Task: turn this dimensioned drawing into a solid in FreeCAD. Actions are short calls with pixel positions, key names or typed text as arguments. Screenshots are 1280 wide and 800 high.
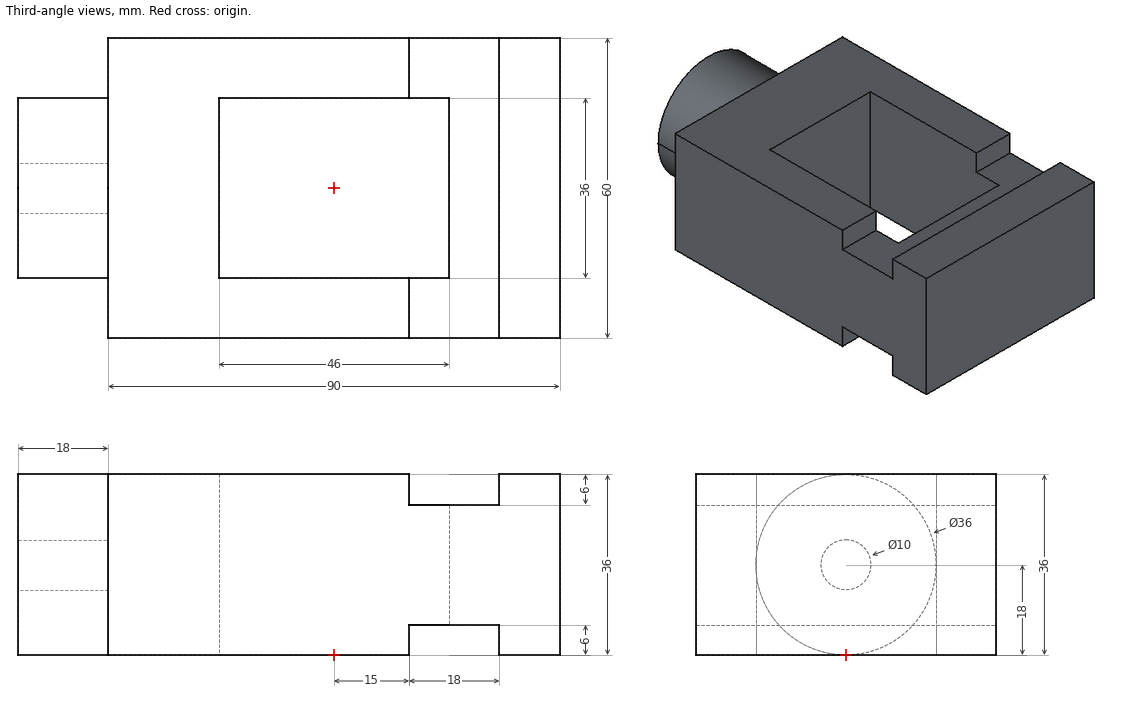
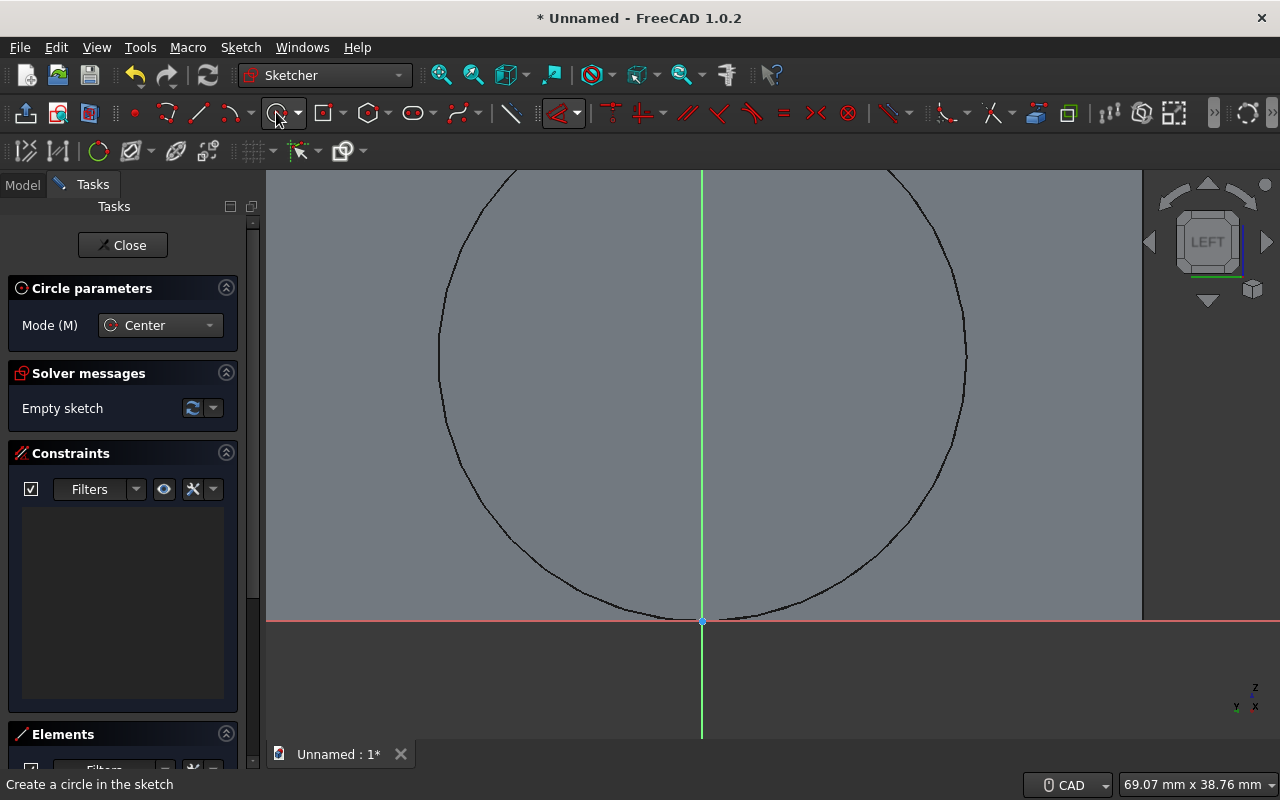
click(702, 357)
click(754, 305)
key(Escape)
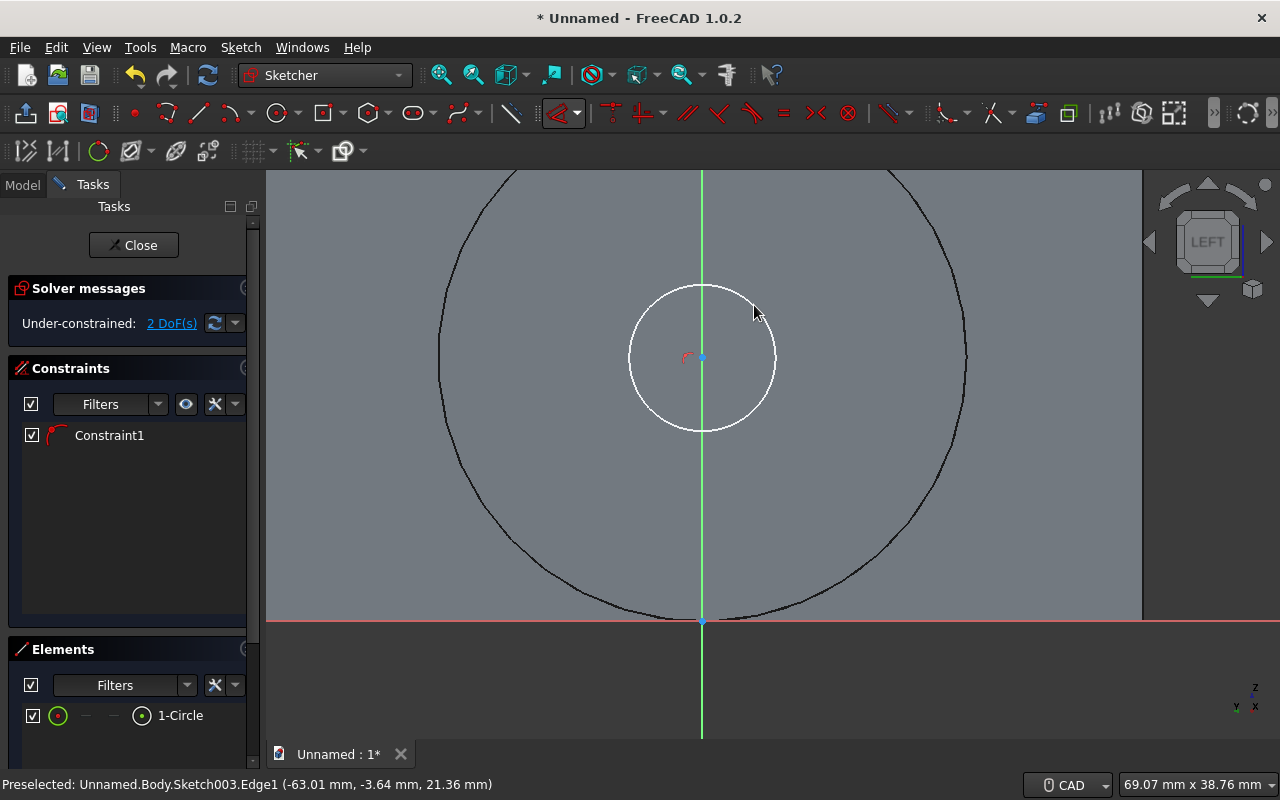
click(754, 306)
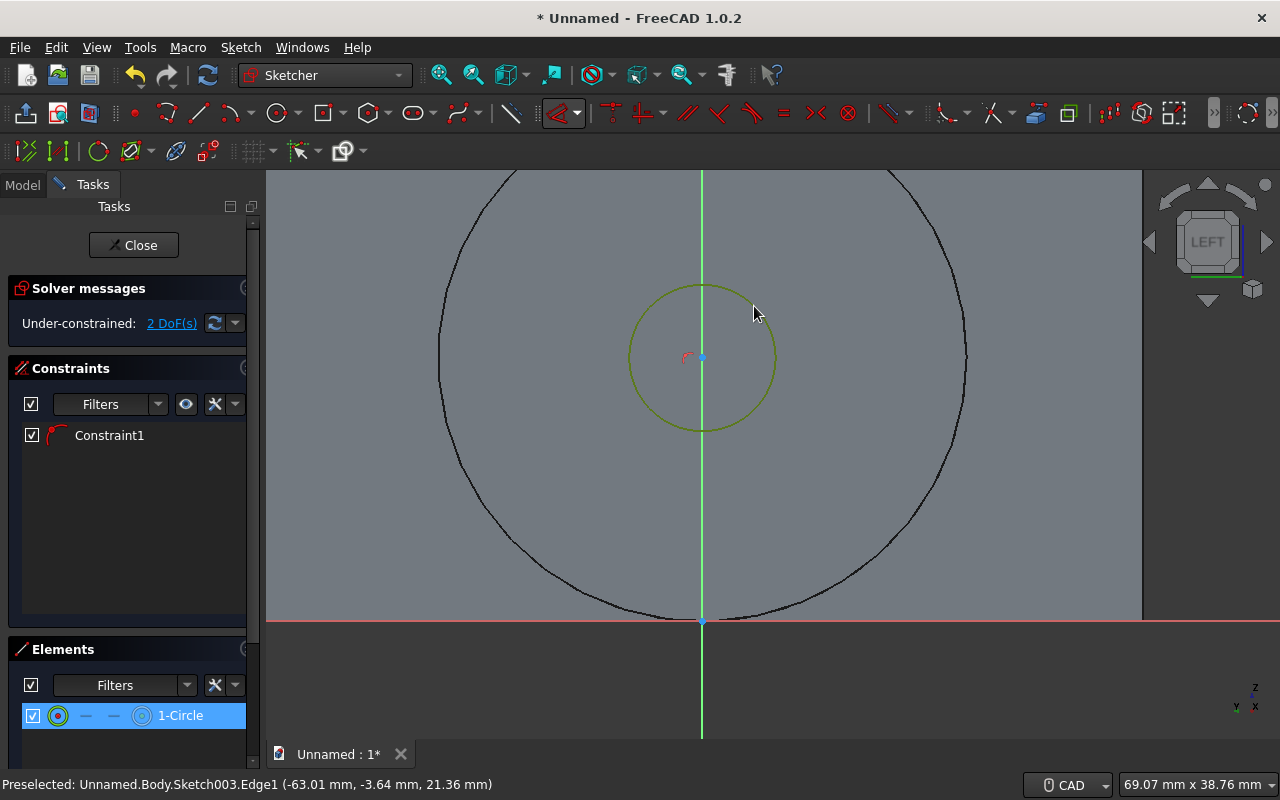
click(580, 114)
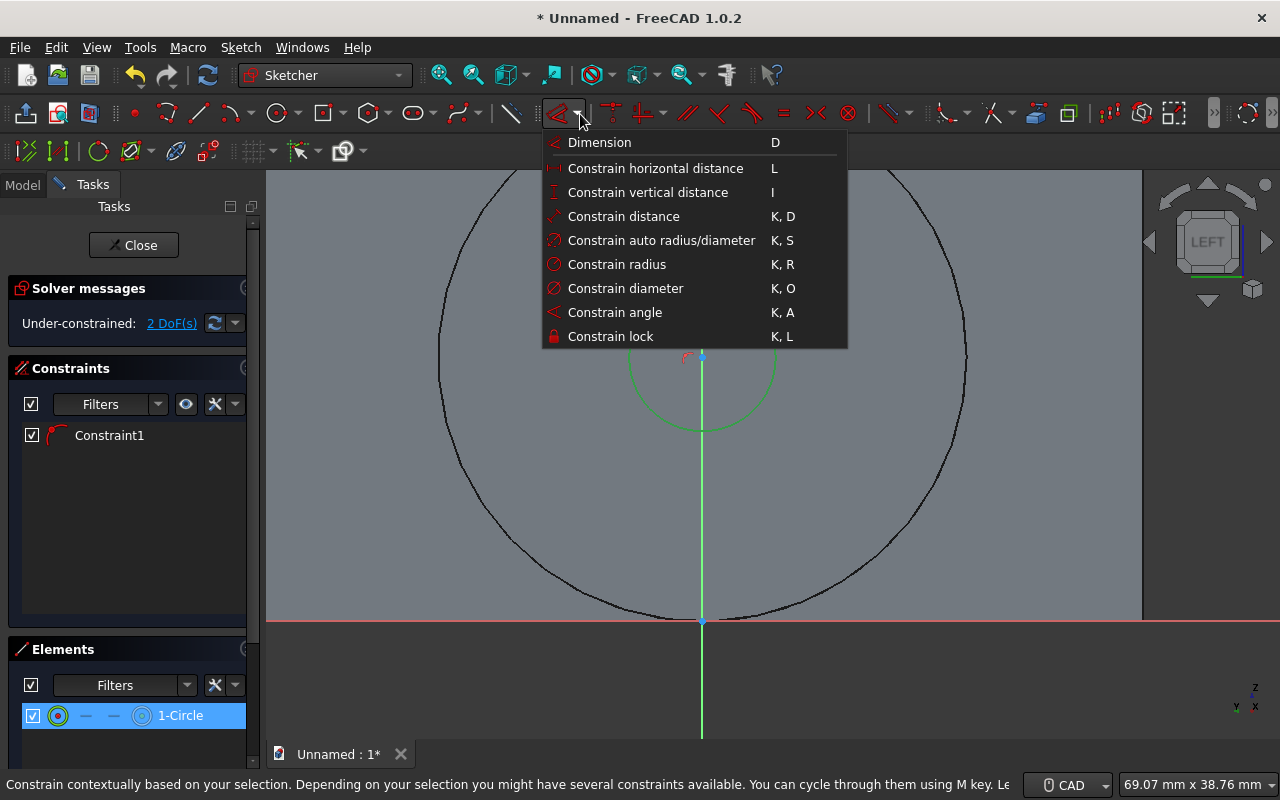
click(695, 288)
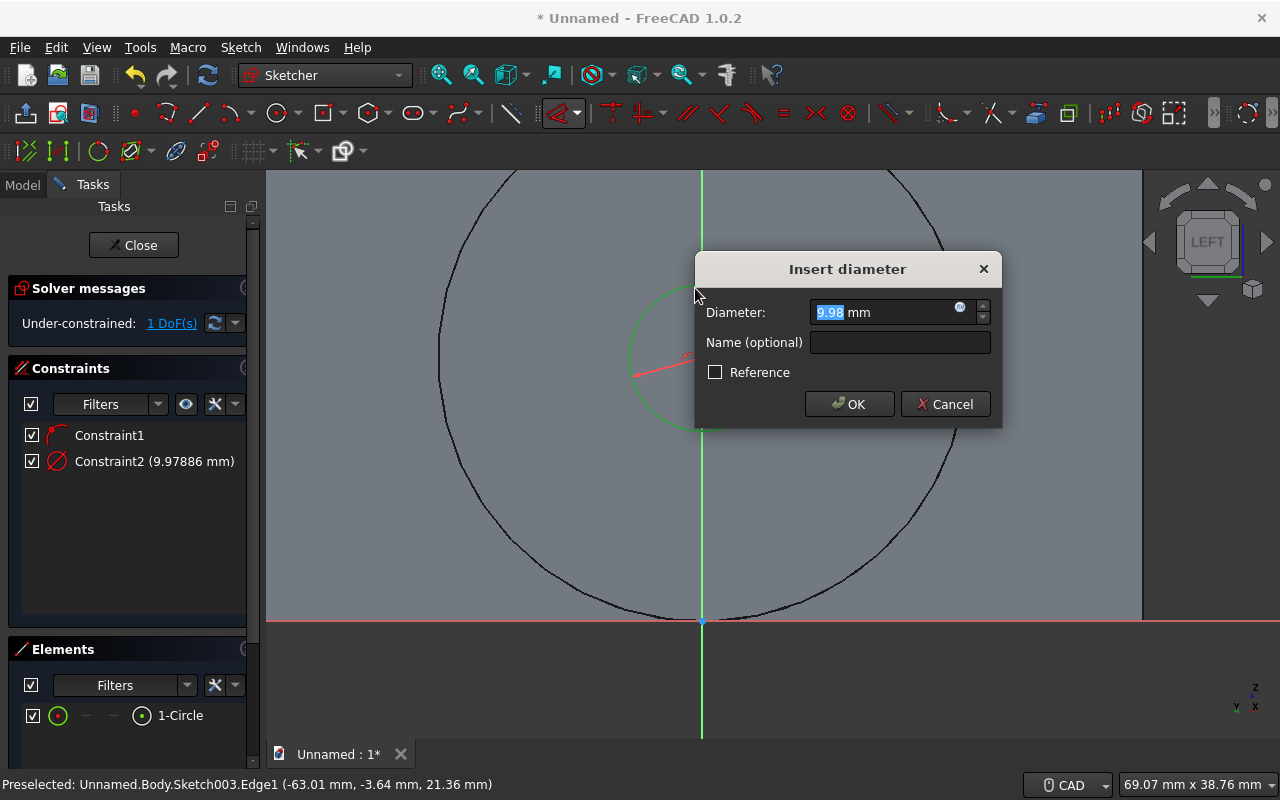
text(10)
key(Return)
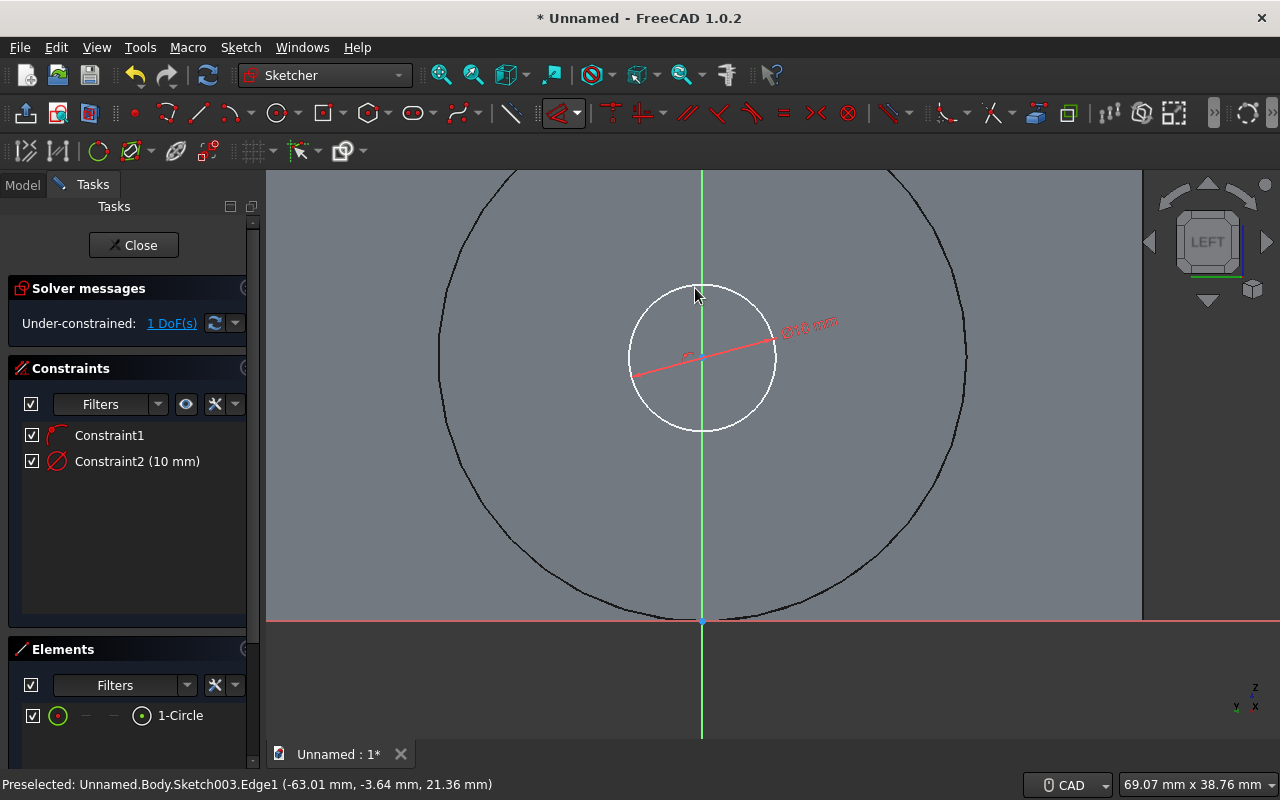
click(702, 358)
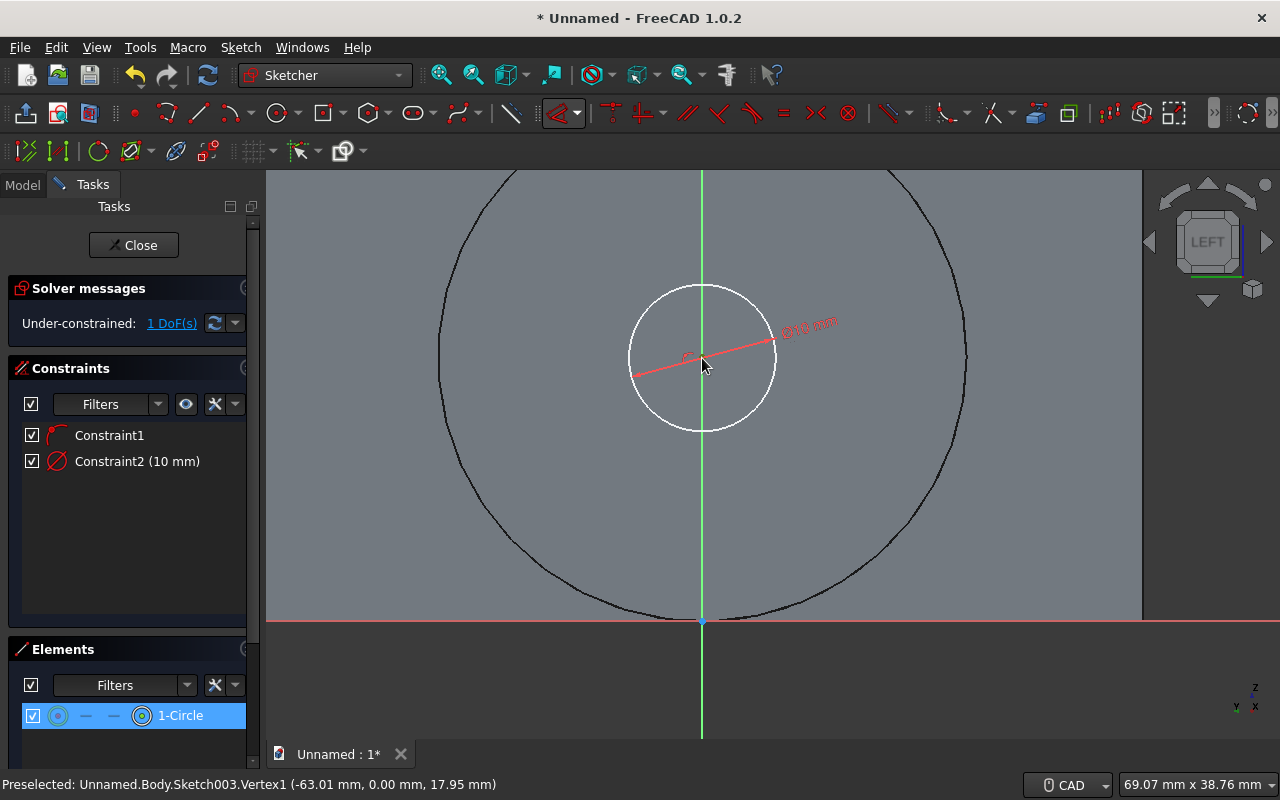
click(580, 114)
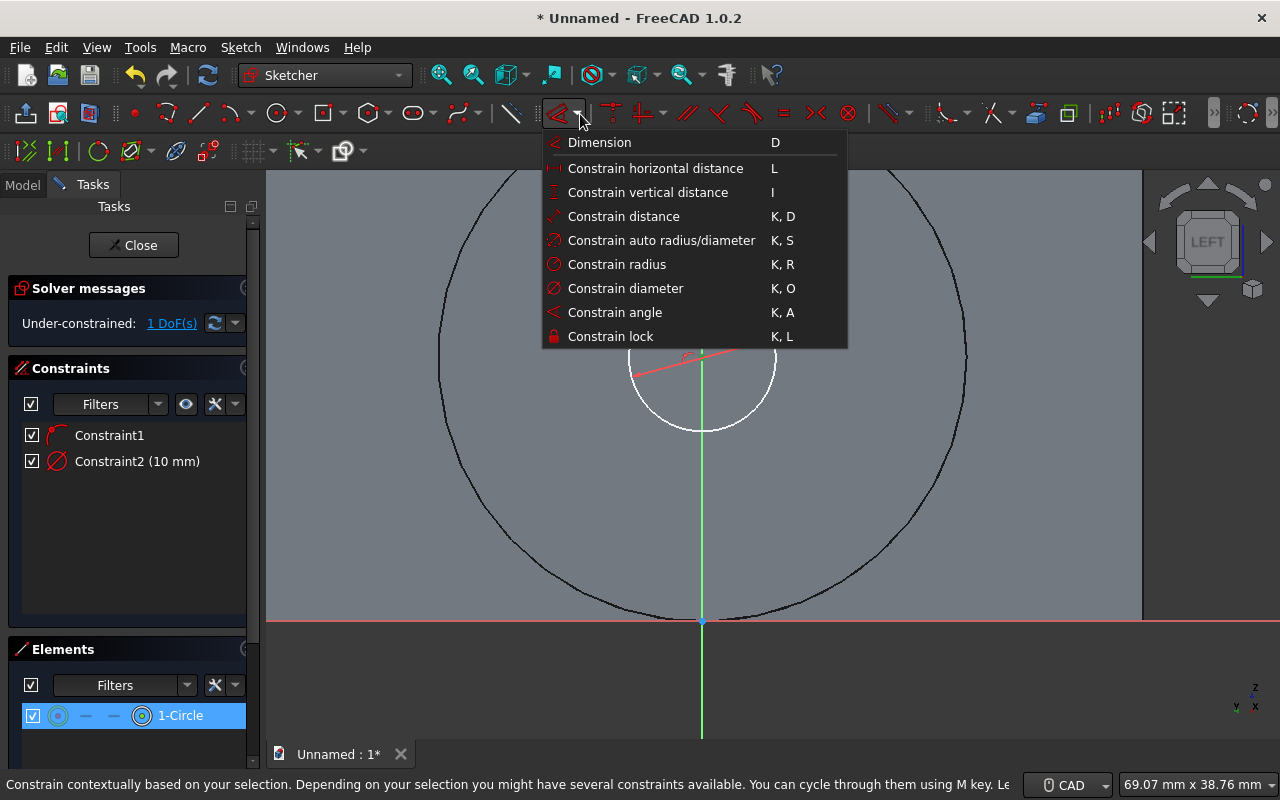
click(695, 192)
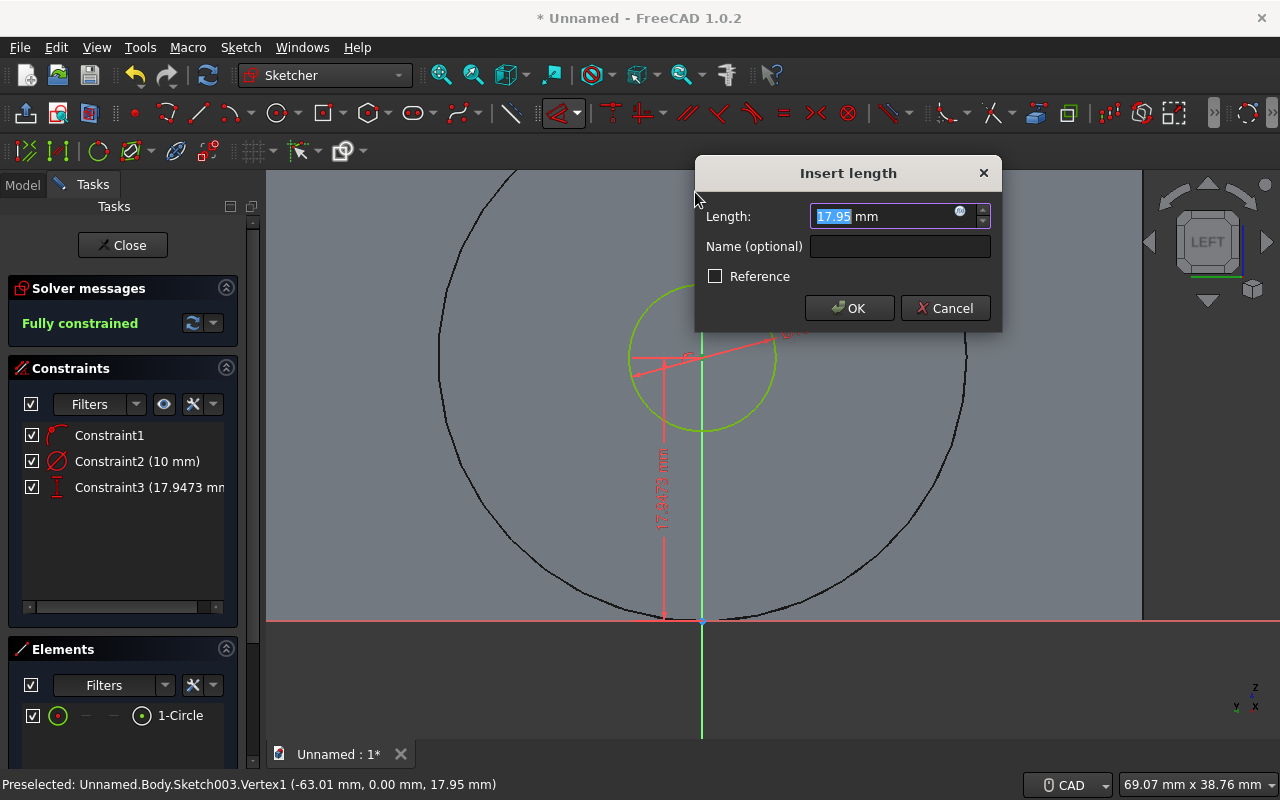
text(18)
key(Return)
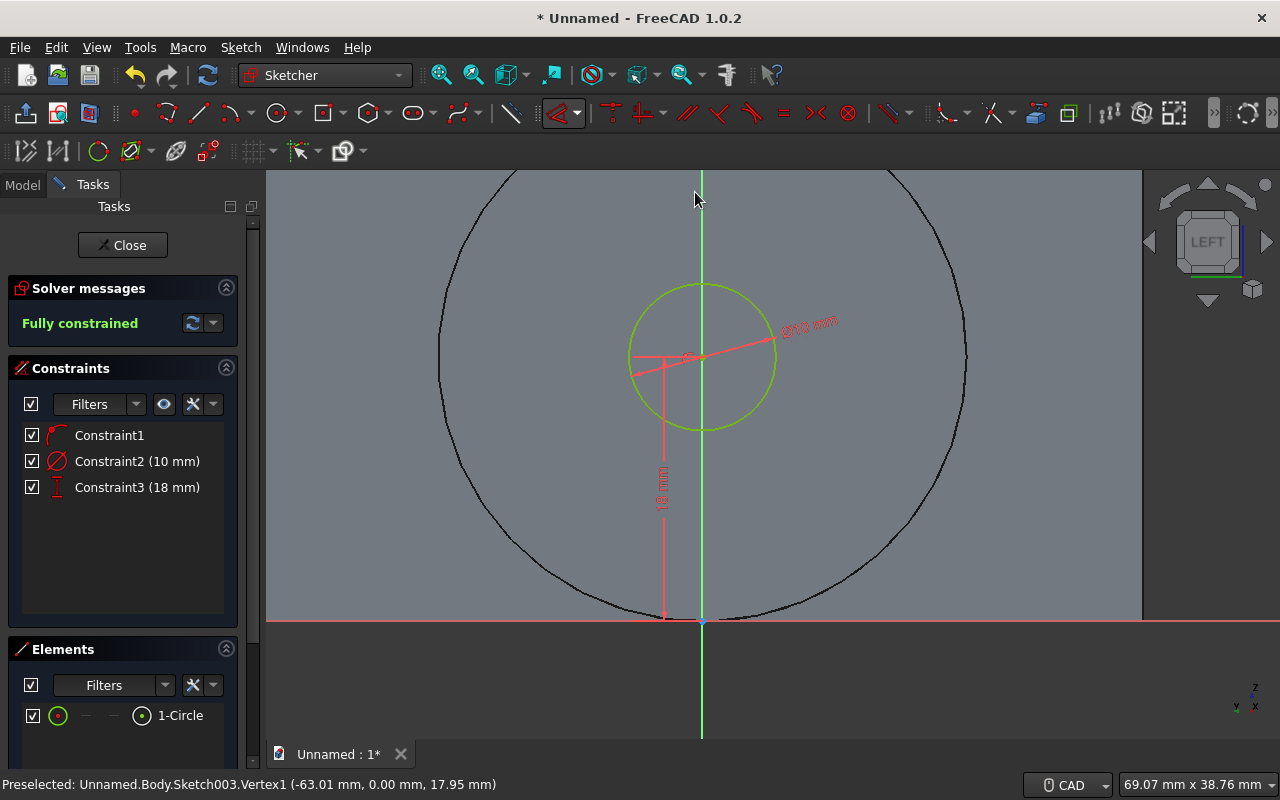
click(123, 245)